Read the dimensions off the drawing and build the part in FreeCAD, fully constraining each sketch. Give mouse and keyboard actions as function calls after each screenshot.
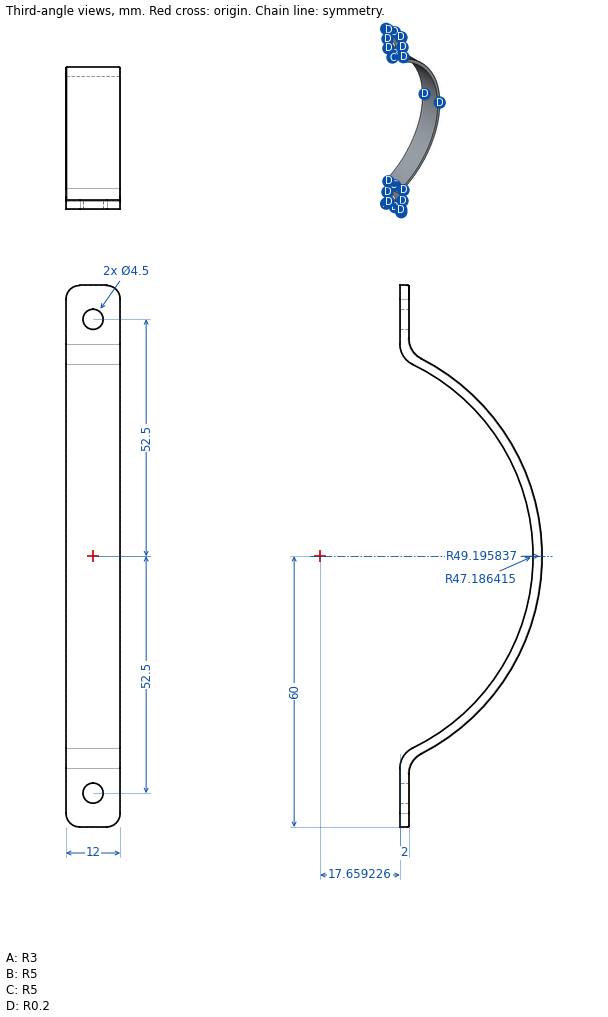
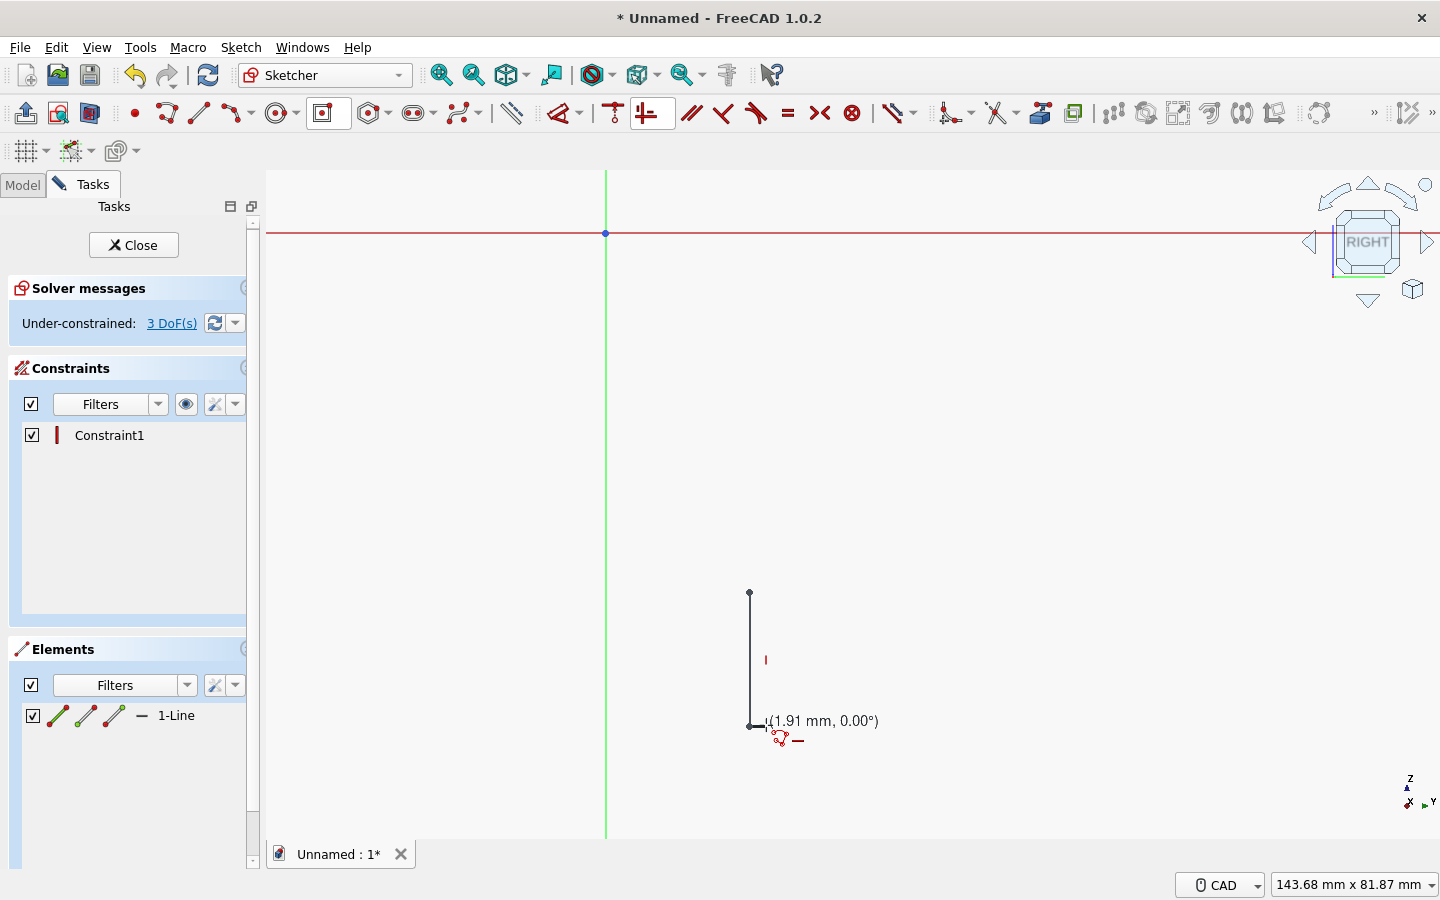
click(766, 724)
click(766, 602)
right_click(766, 602)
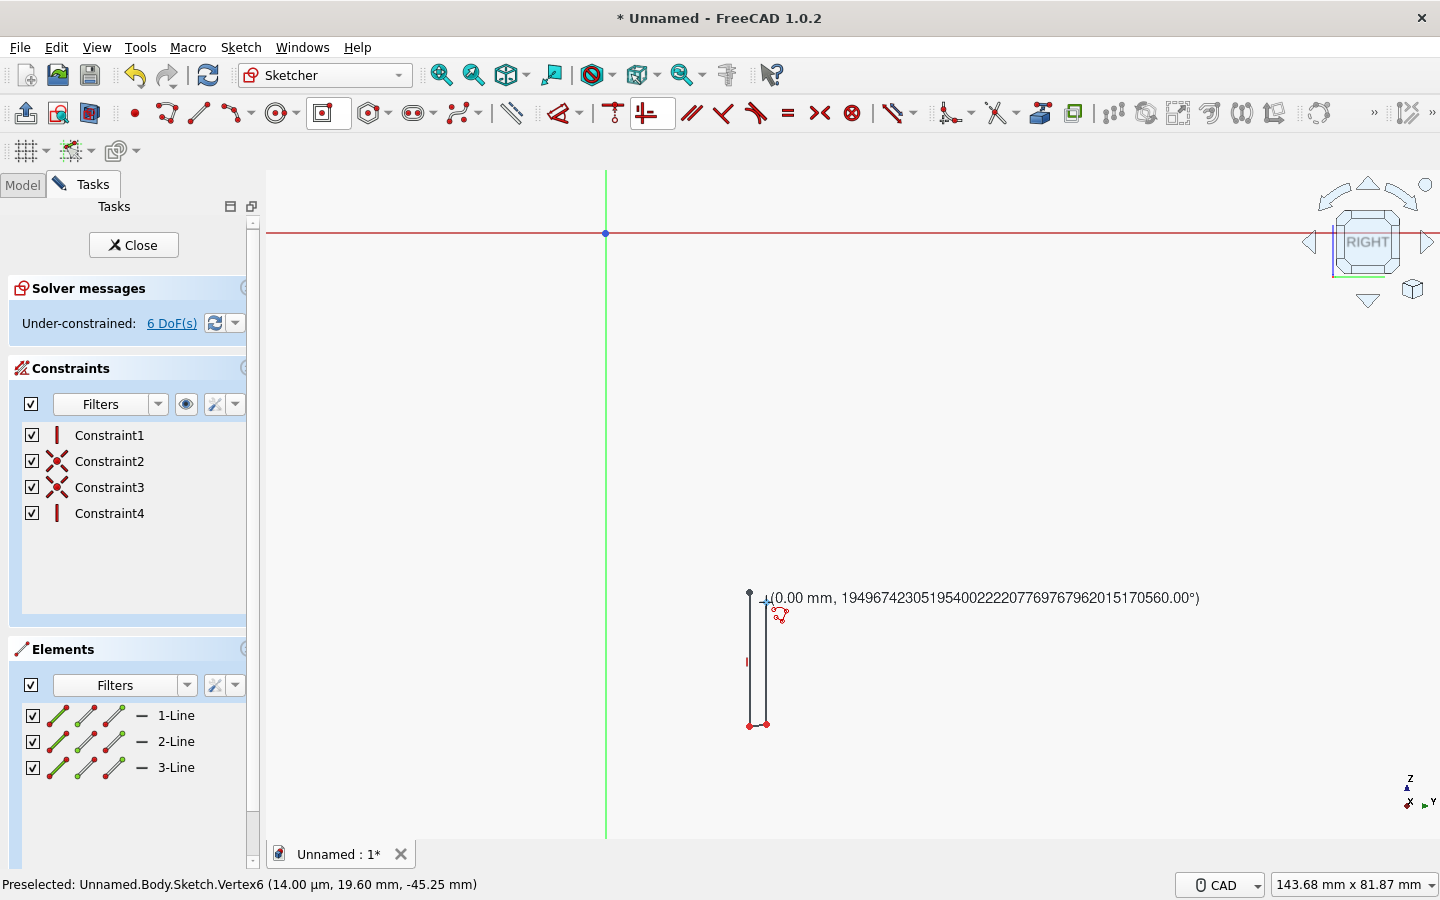
scroll(766, 726, down, 4)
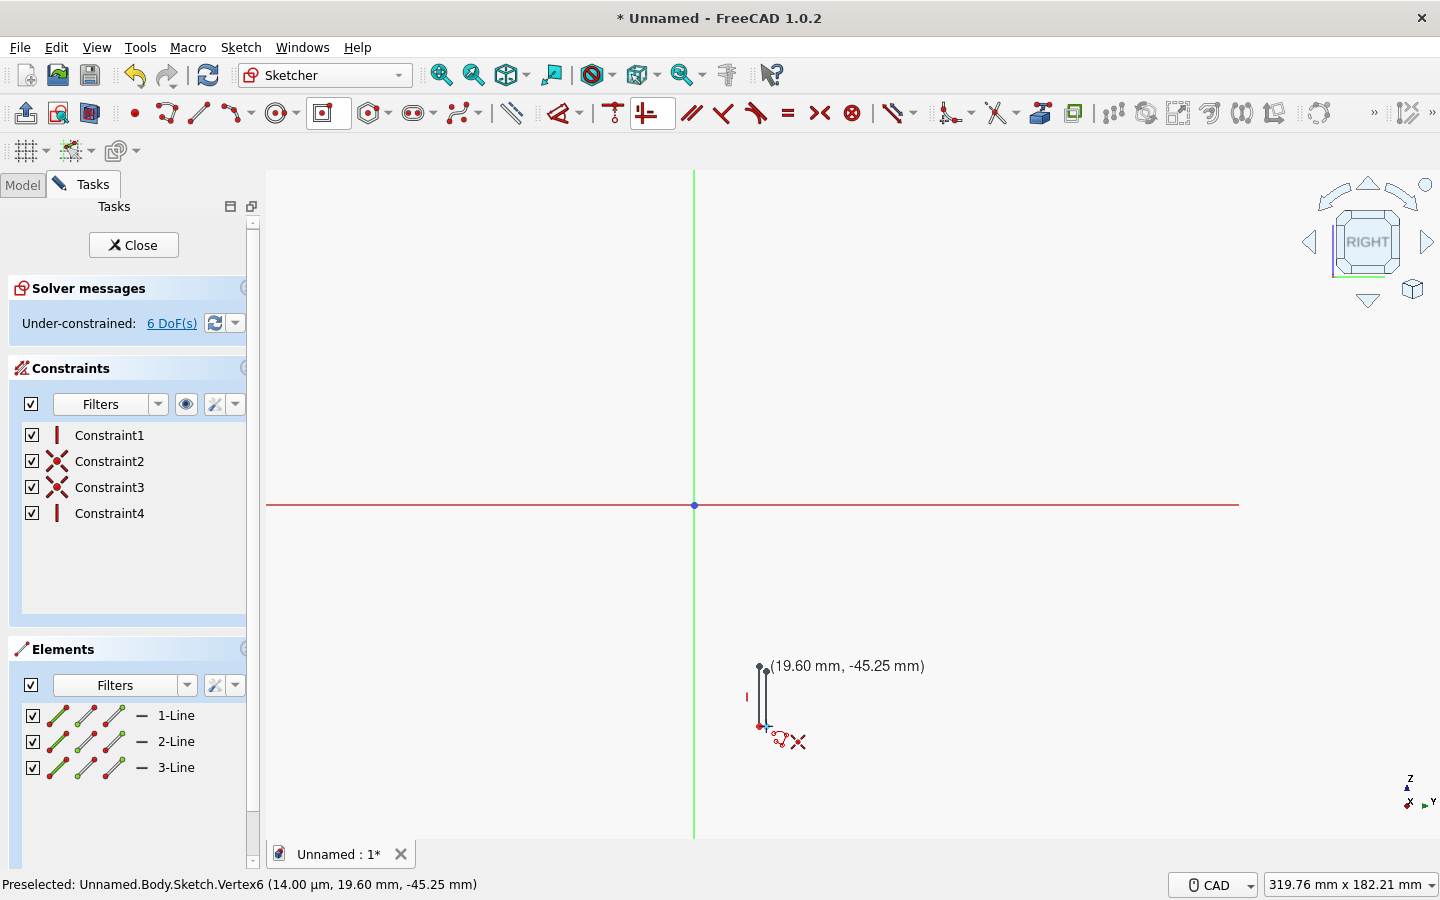
click(766, 339)
click(766, 285)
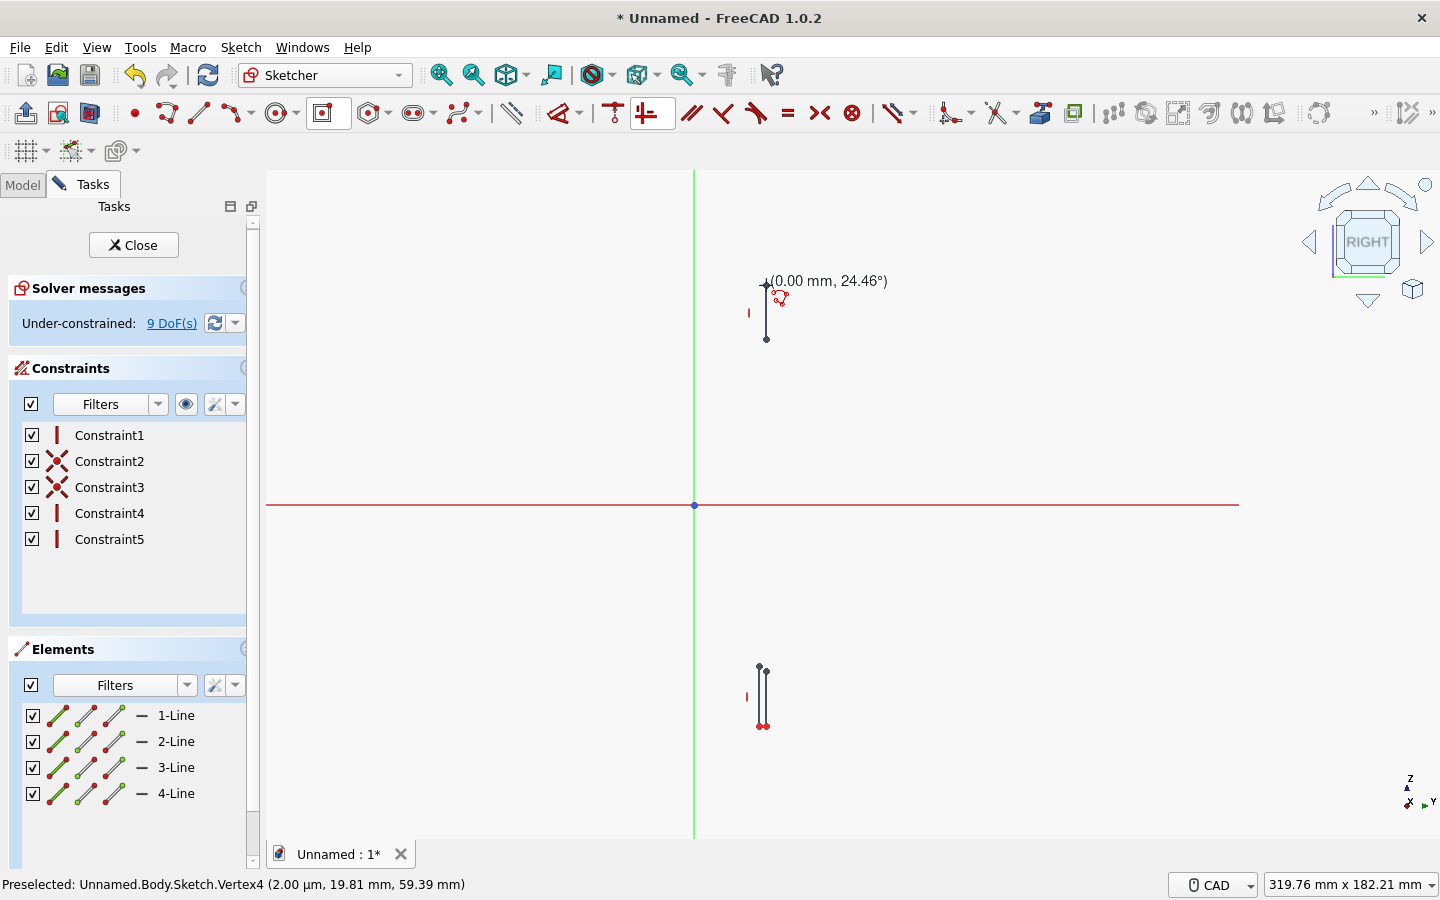
scroll(759, 285, up, 4)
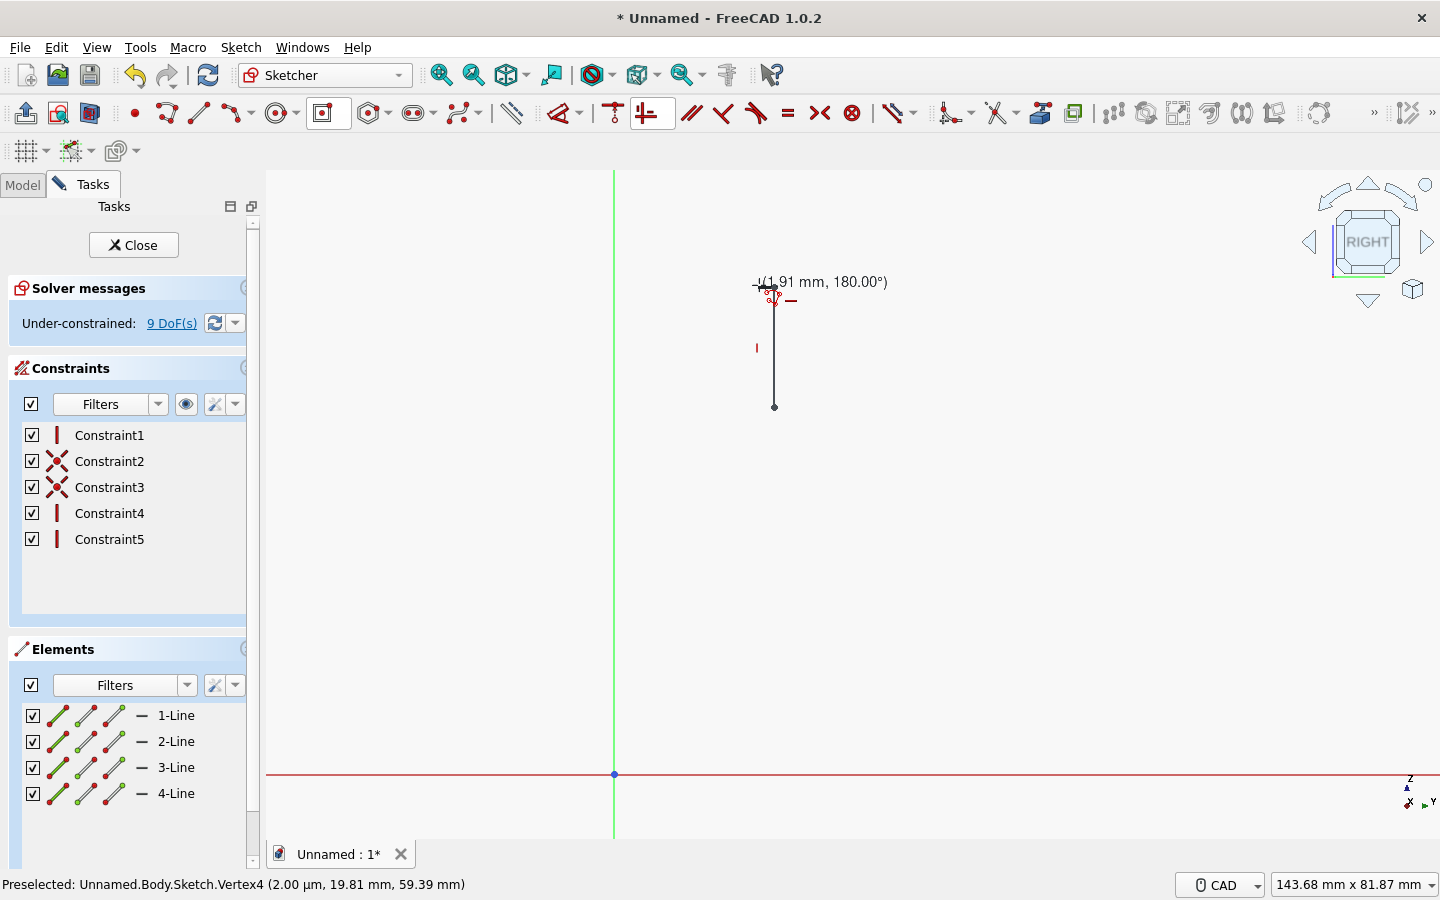
click(759, 285)
click(759, 417)
right_click(759, 417)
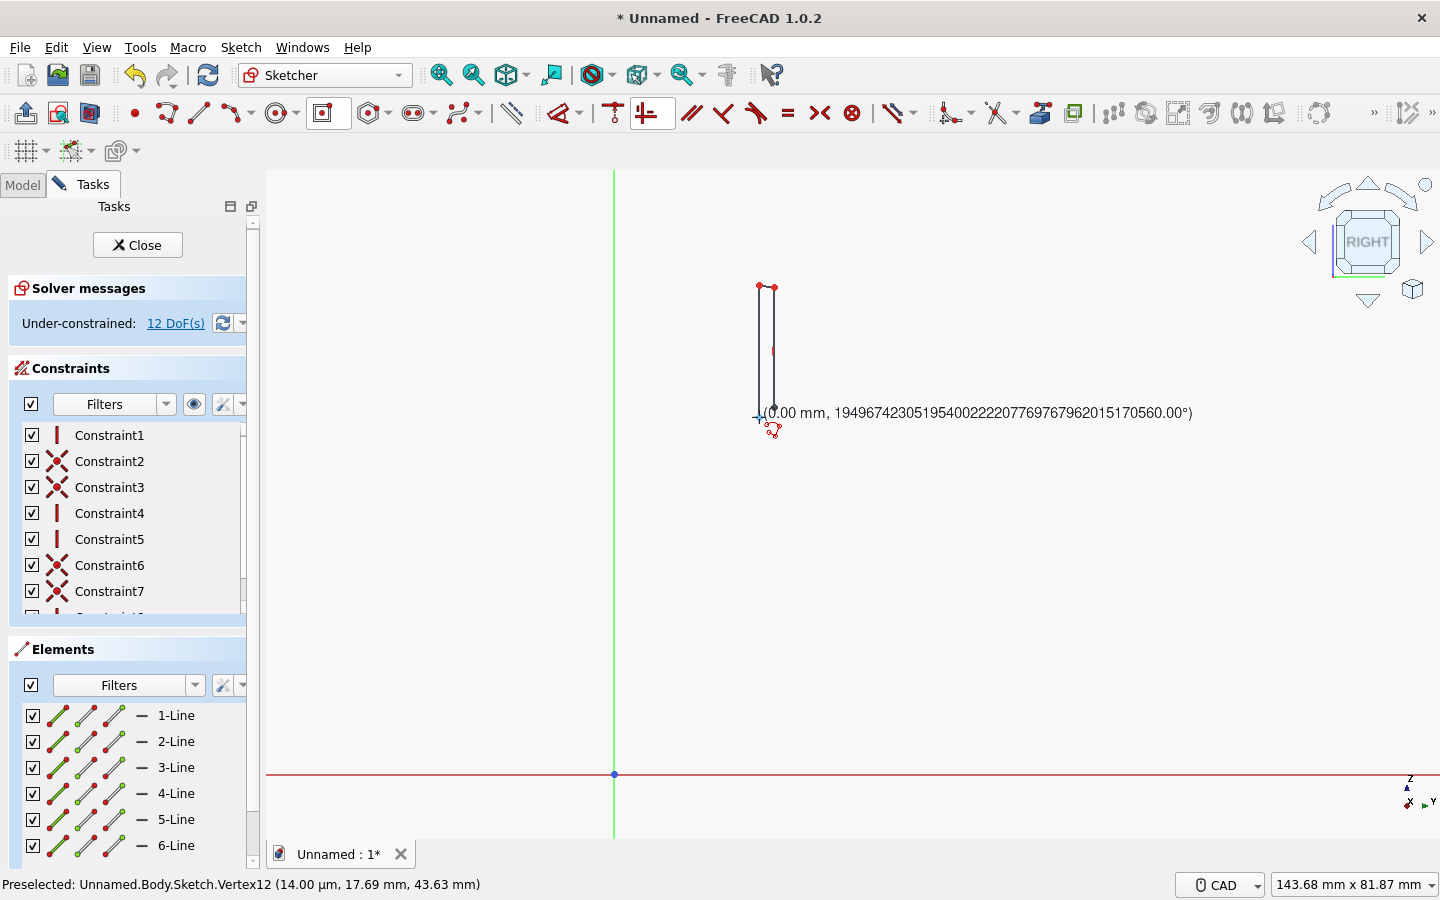
click(232, 114)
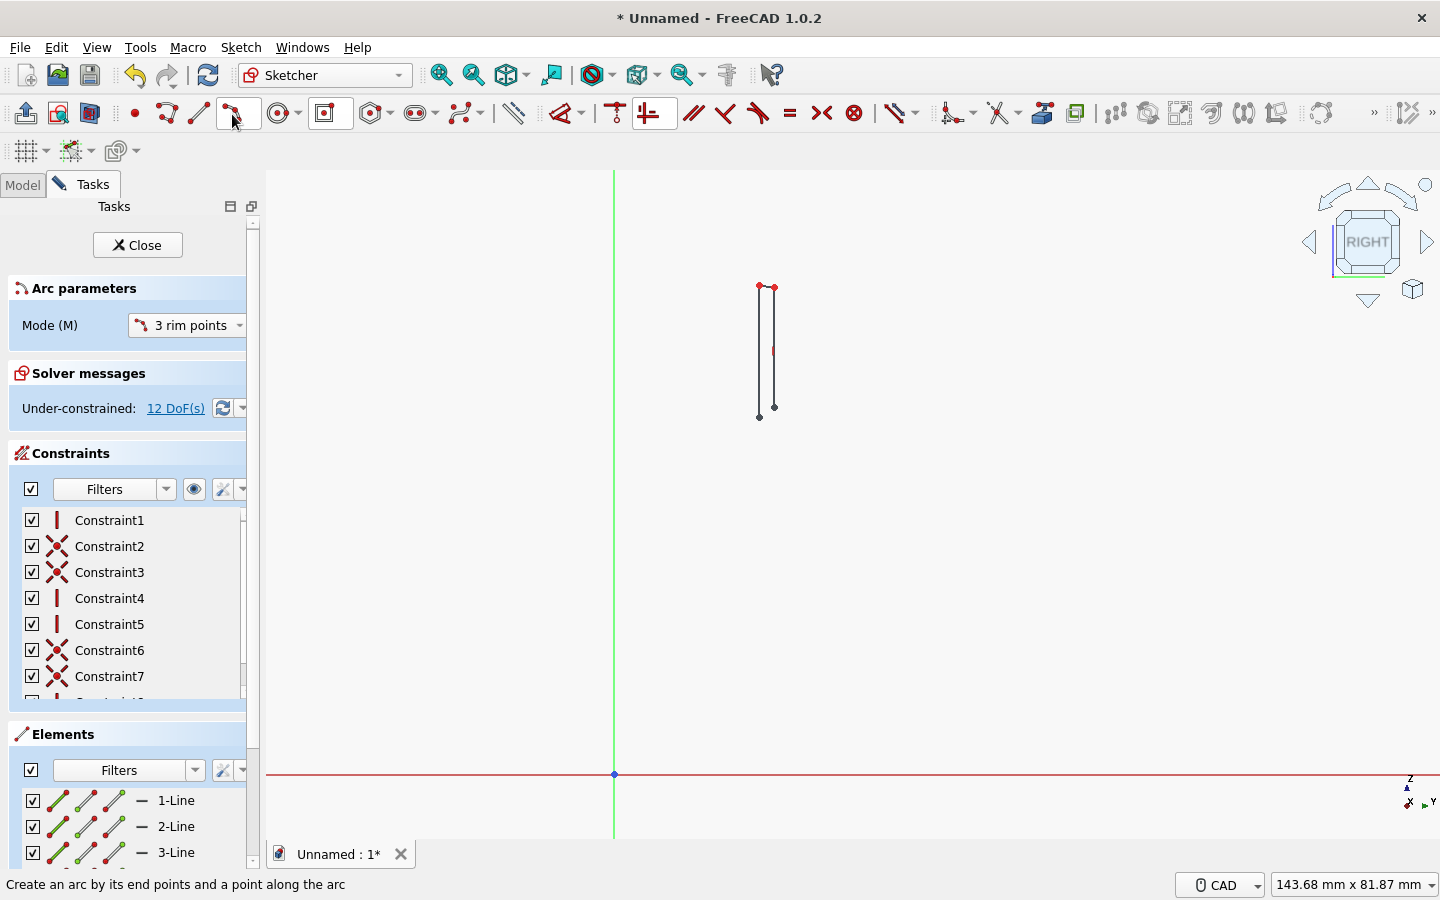
scroll(759, 284, down, 4)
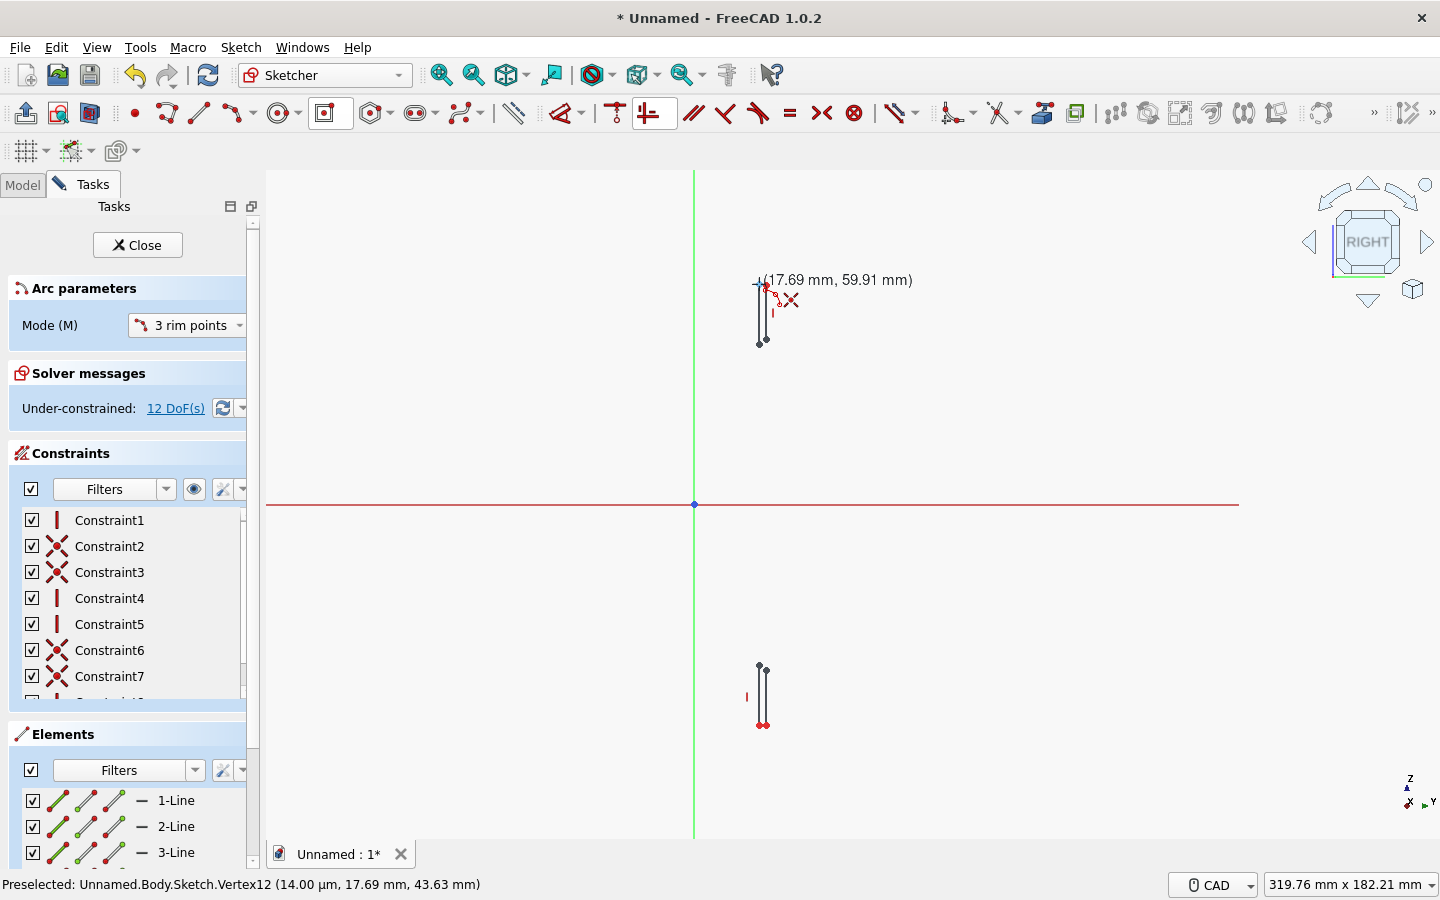
scroll(766, 670, up, 4)